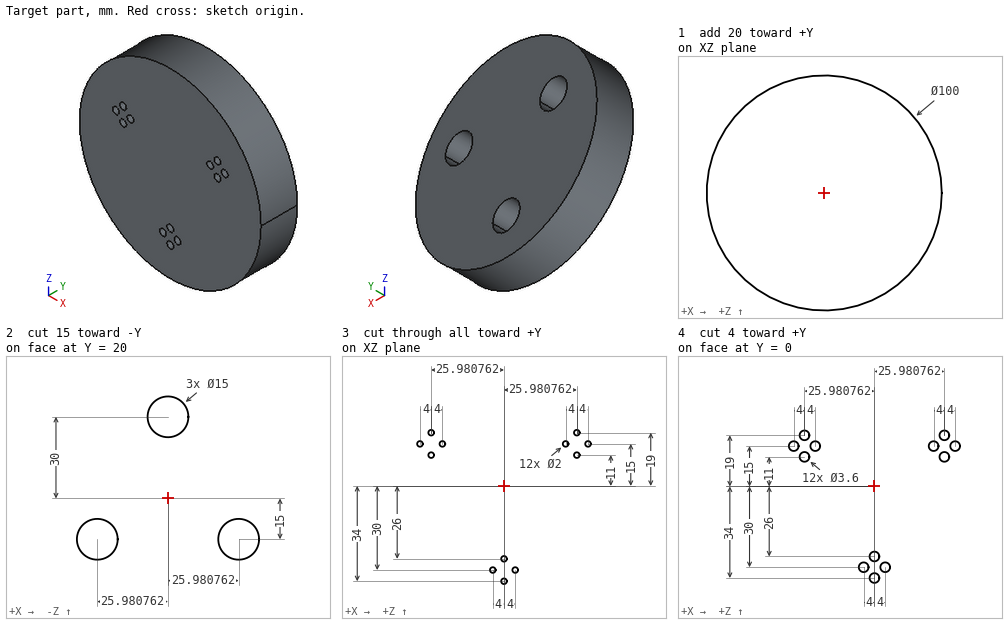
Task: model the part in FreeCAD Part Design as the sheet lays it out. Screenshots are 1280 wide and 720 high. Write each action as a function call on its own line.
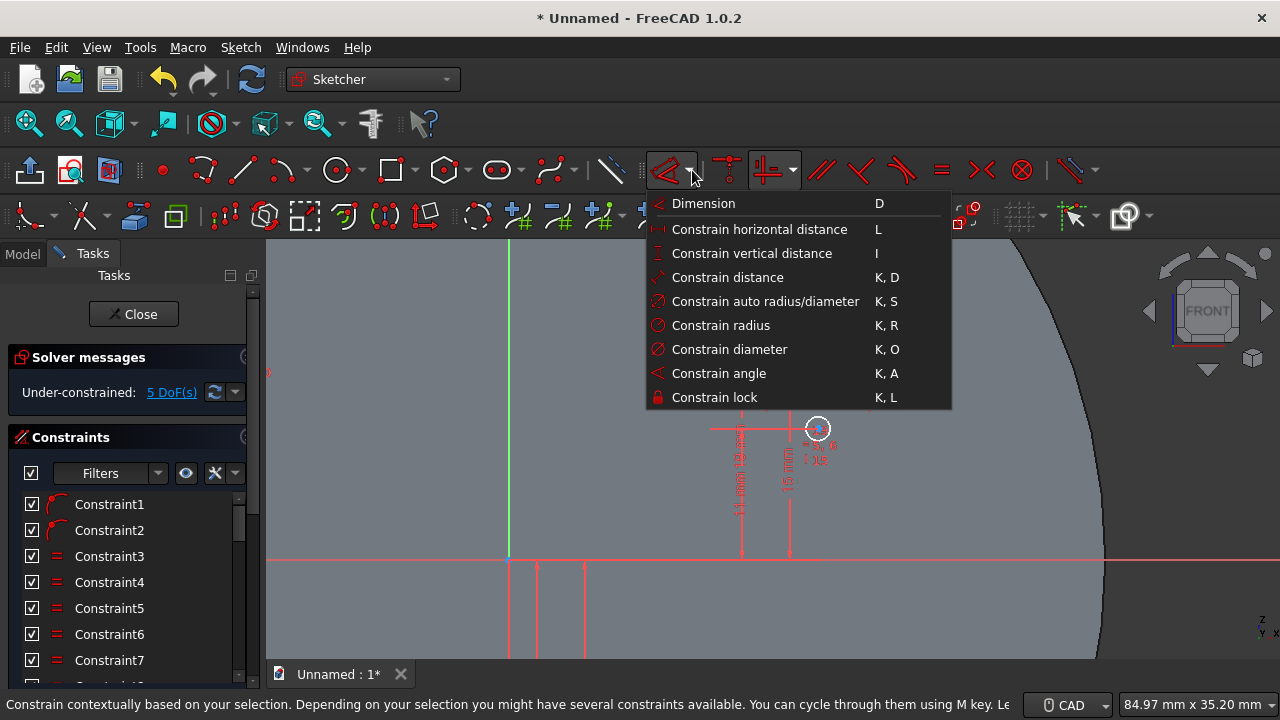
click(799, 229)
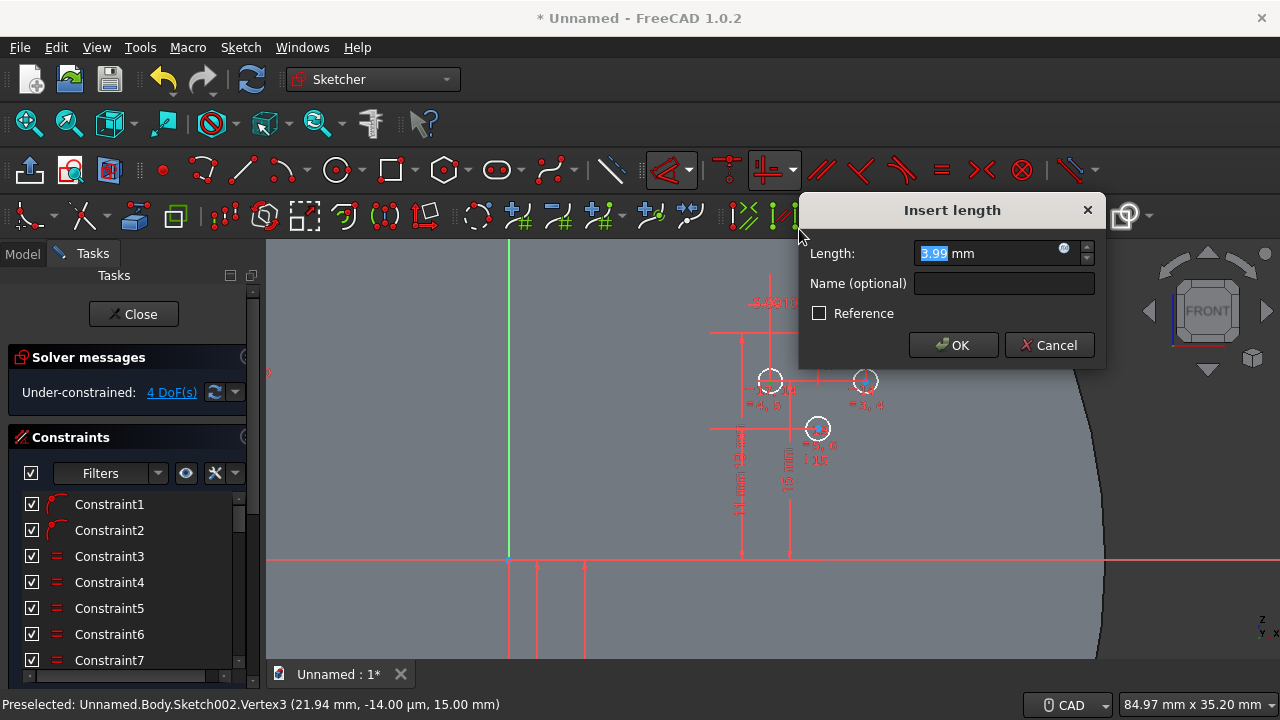
text(4)
key(Return)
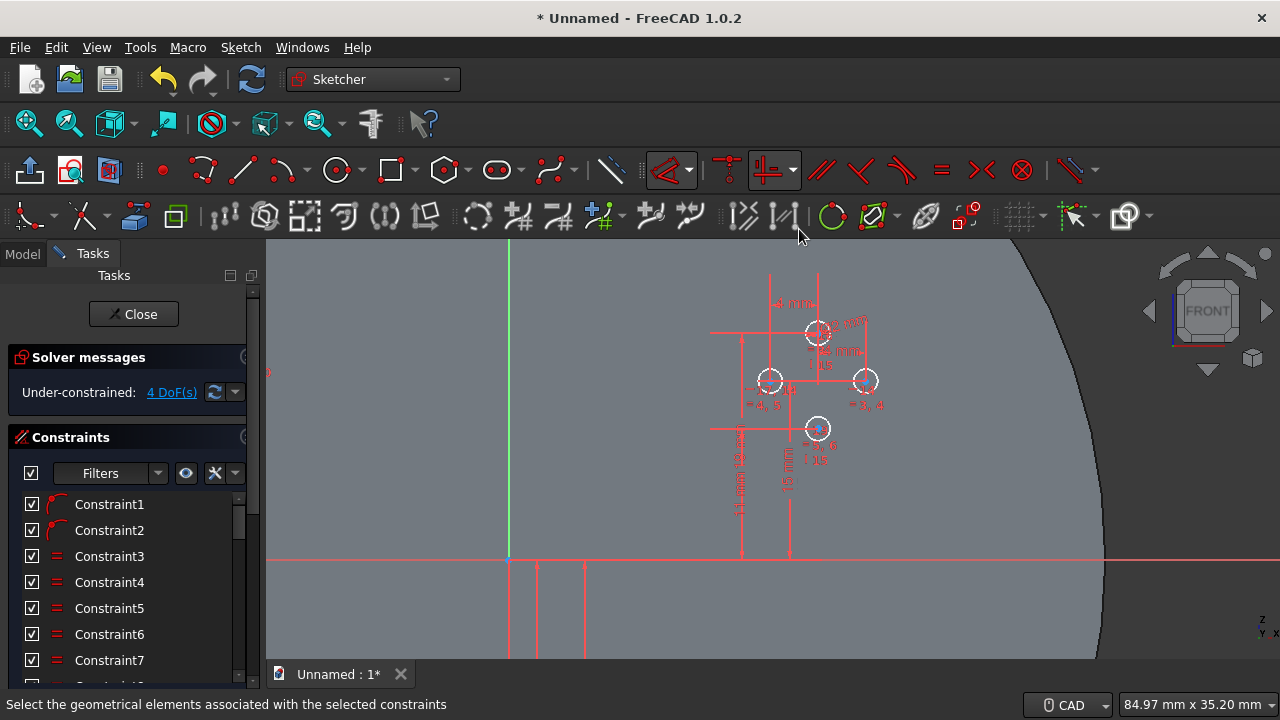
scroll(818, 332, down, 5)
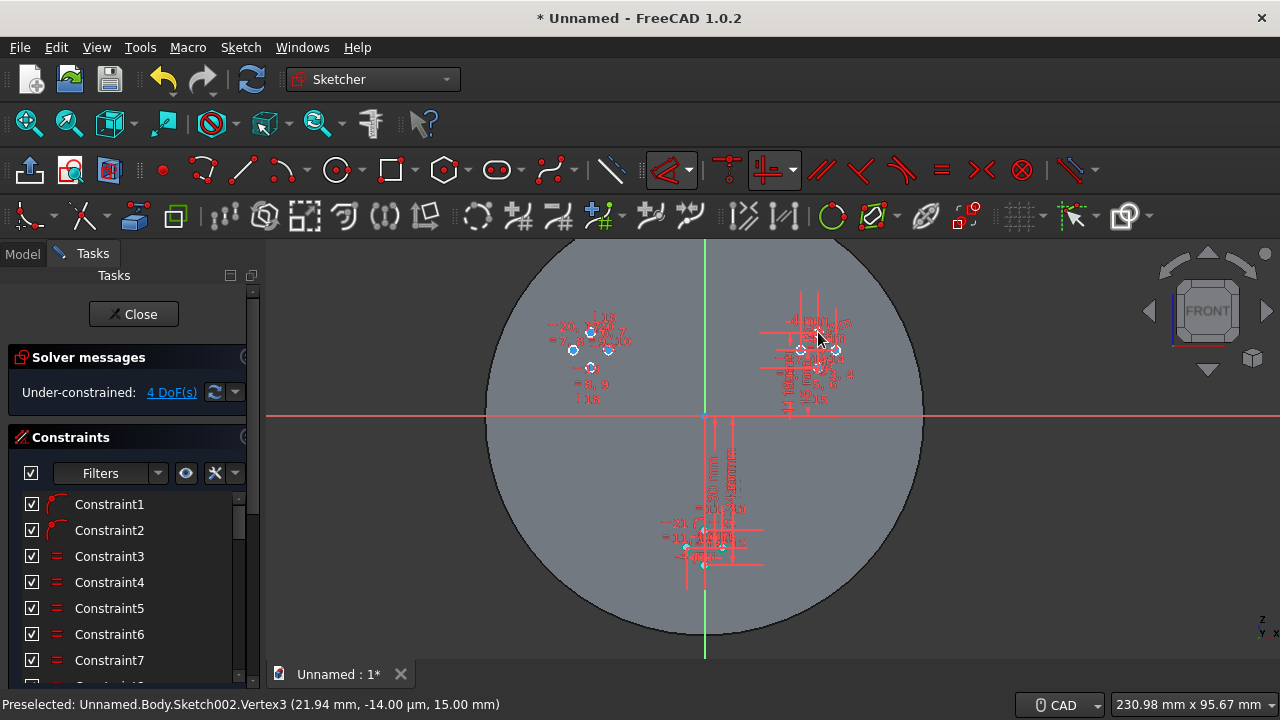
scroll(591, 333, up, 5)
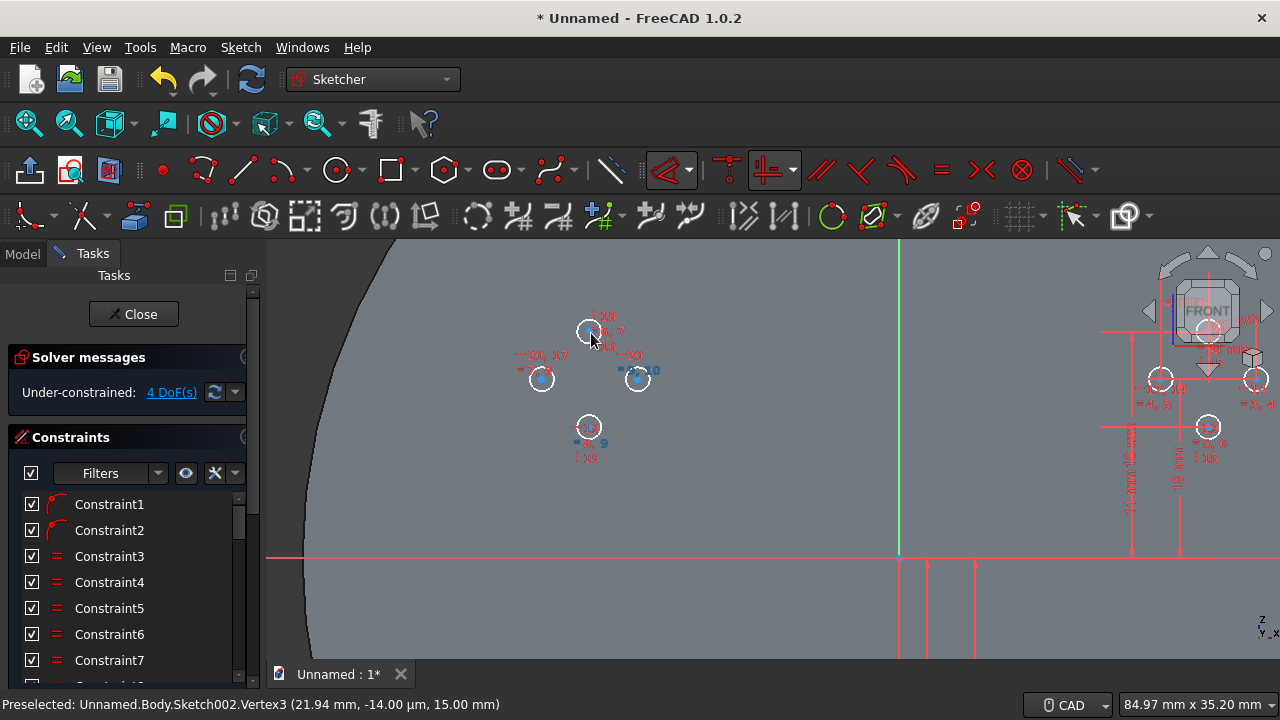
click(589, 332)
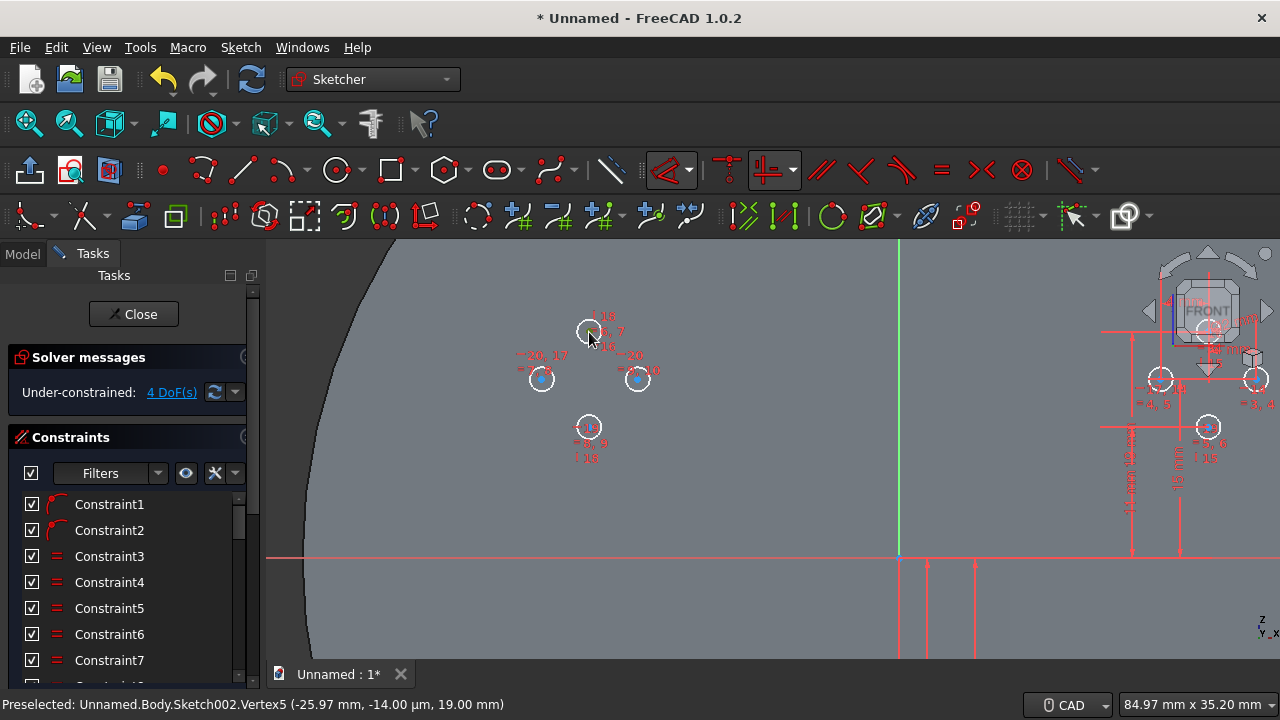
click(542, 379)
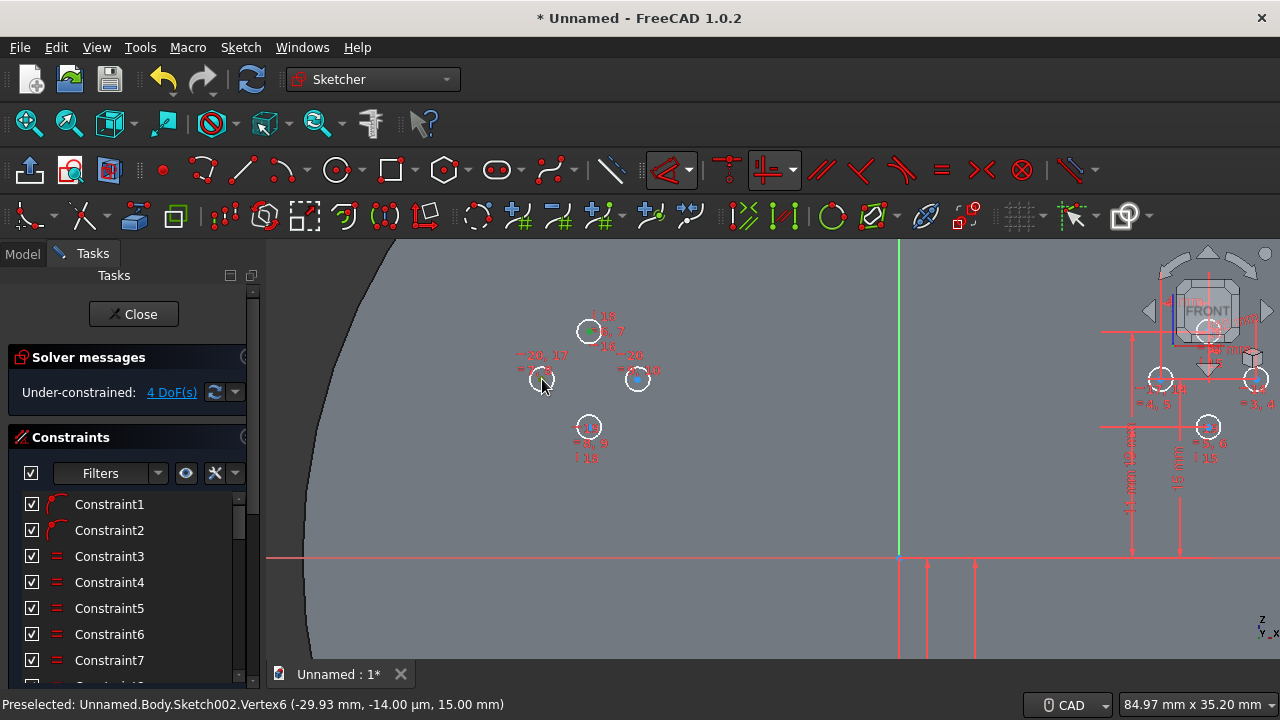
key(l)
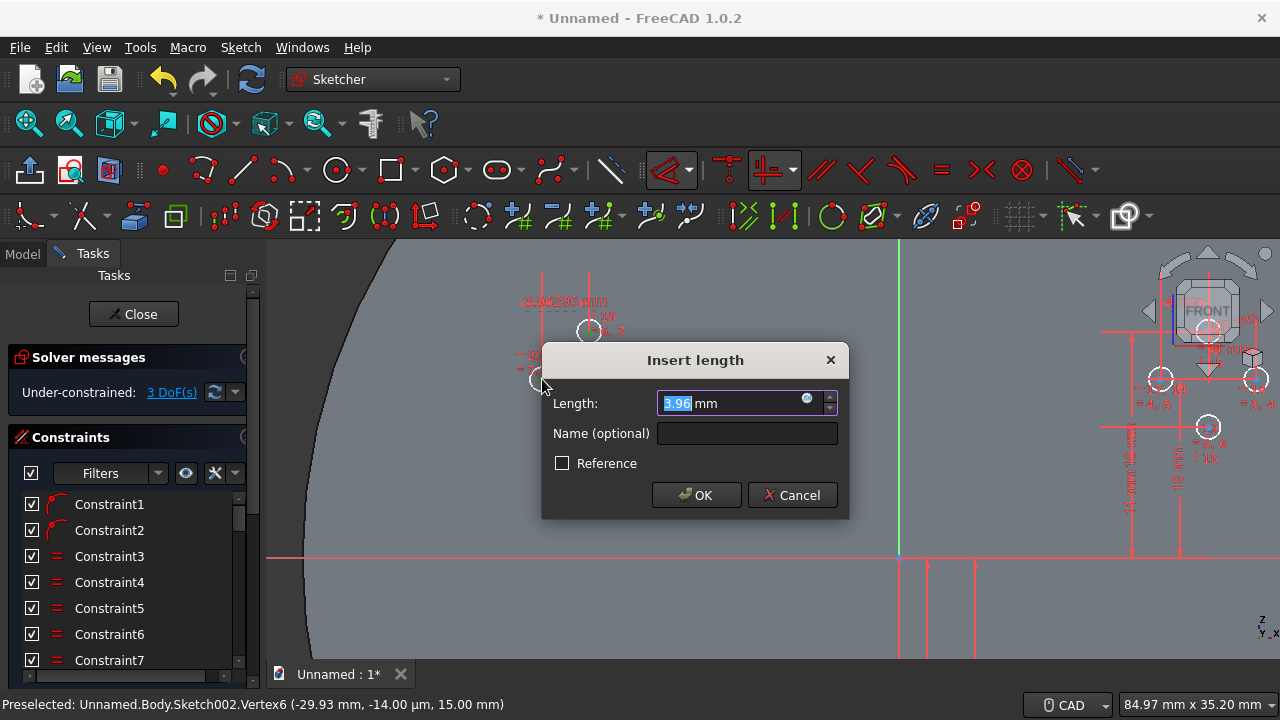
text(4)
key(Return)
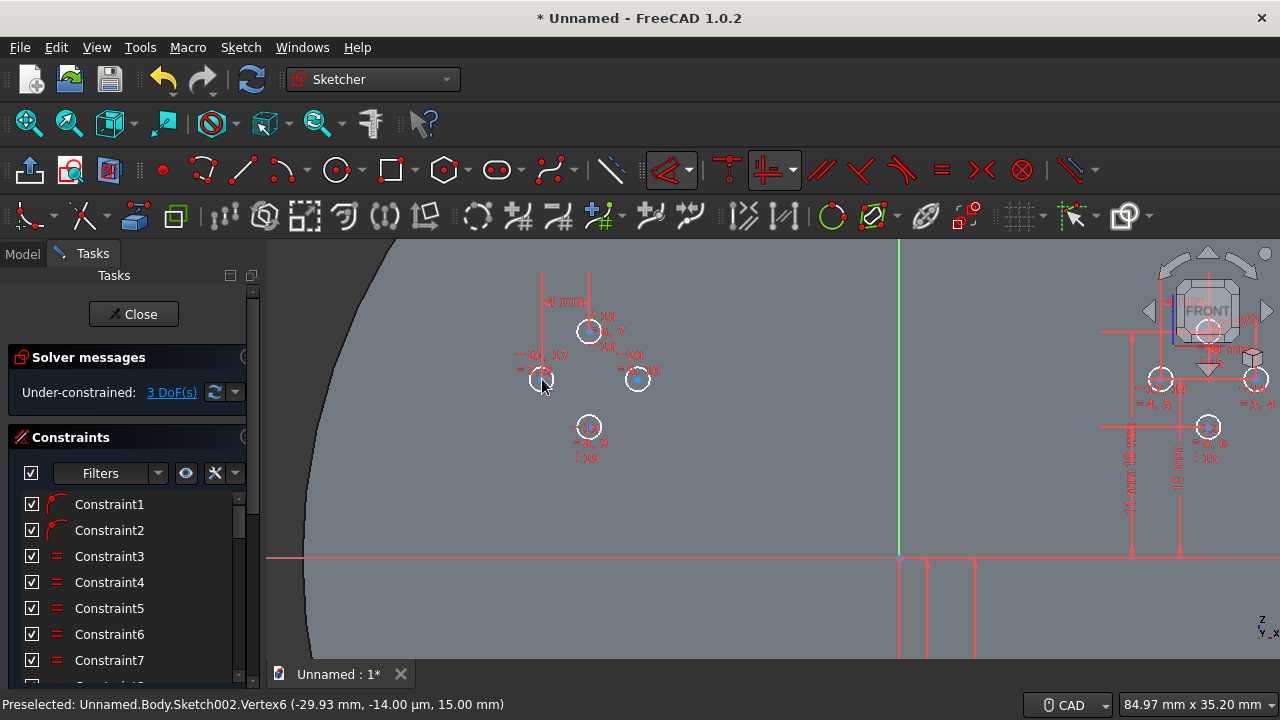
click(589, 332)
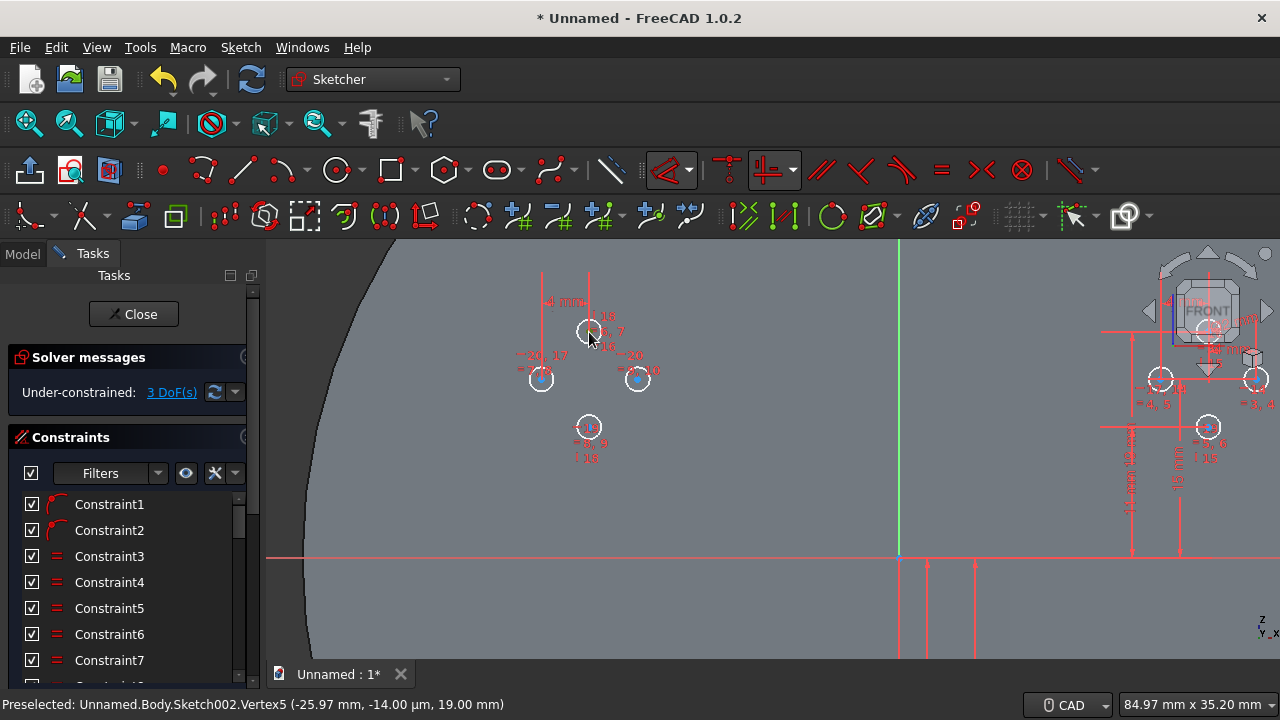
click(638, 379)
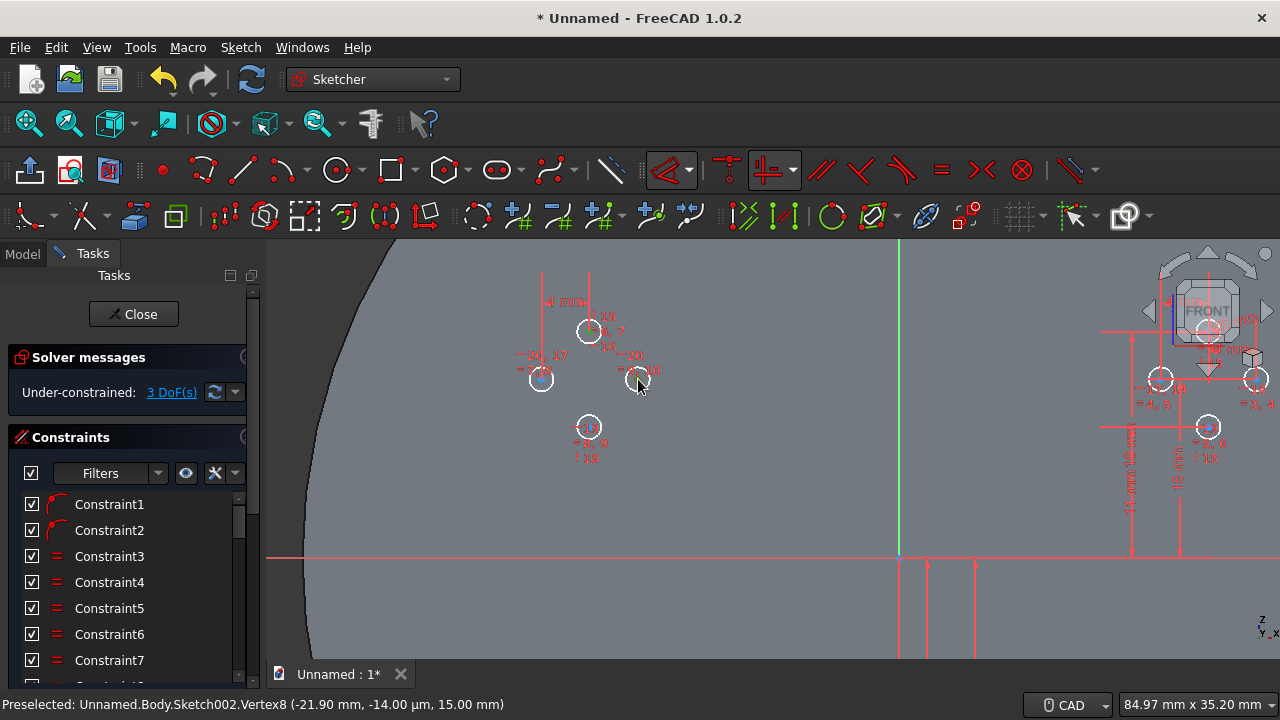
key(l)